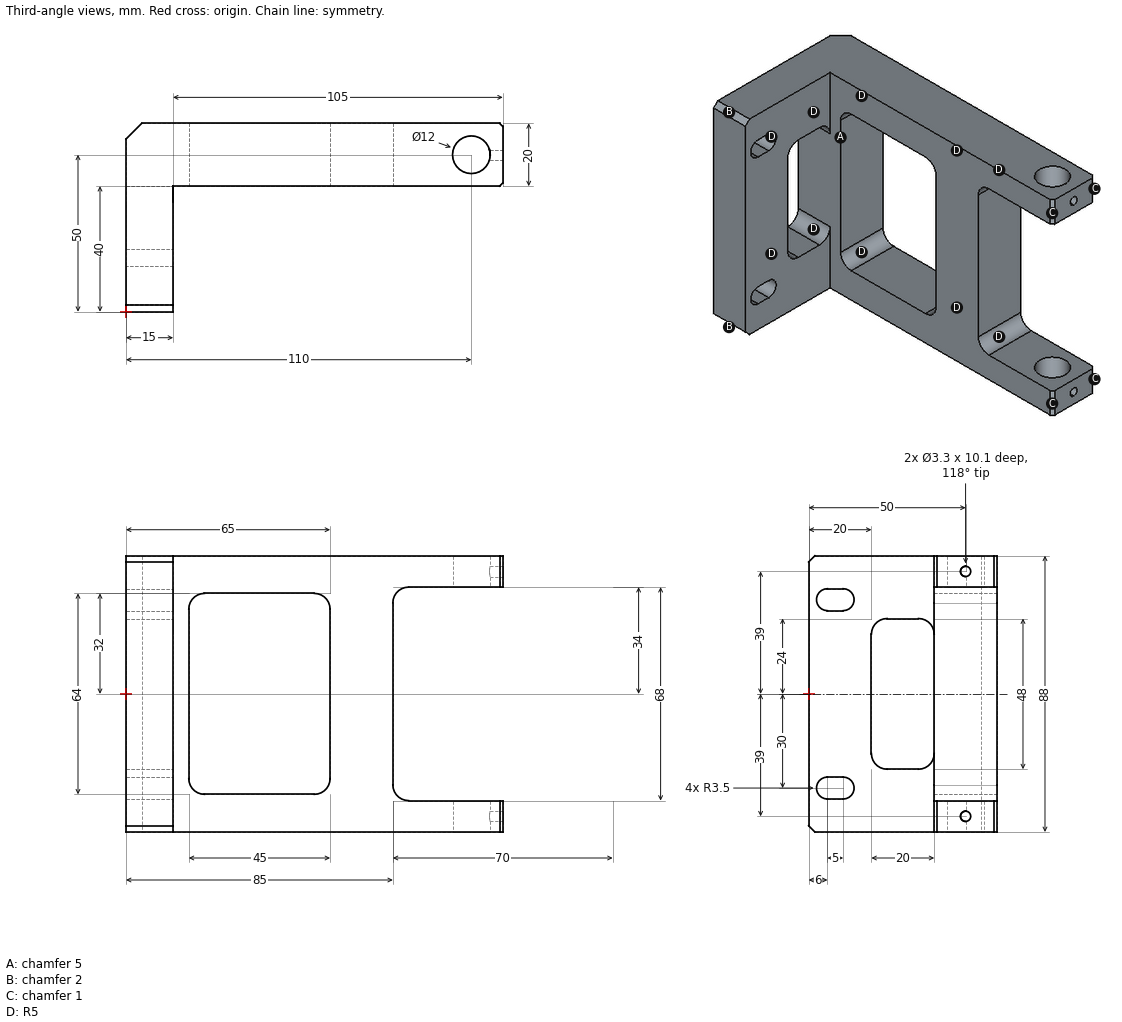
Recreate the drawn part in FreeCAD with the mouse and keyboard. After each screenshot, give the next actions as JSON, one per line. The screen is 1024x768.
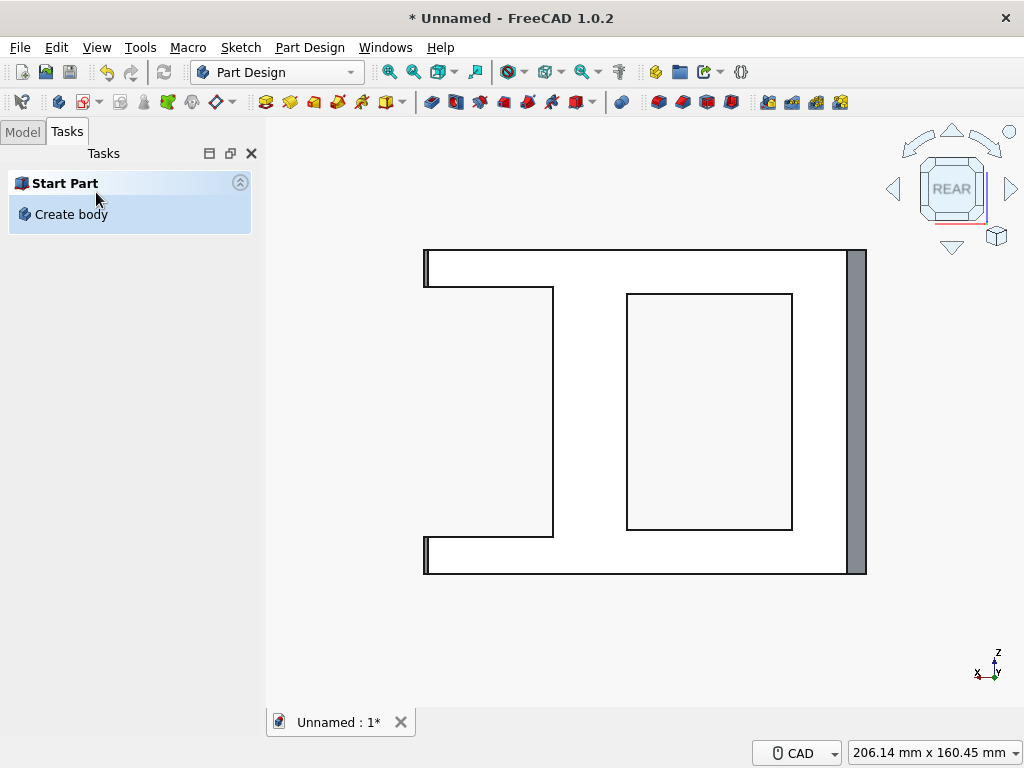
{"action": "key", "text": "6"}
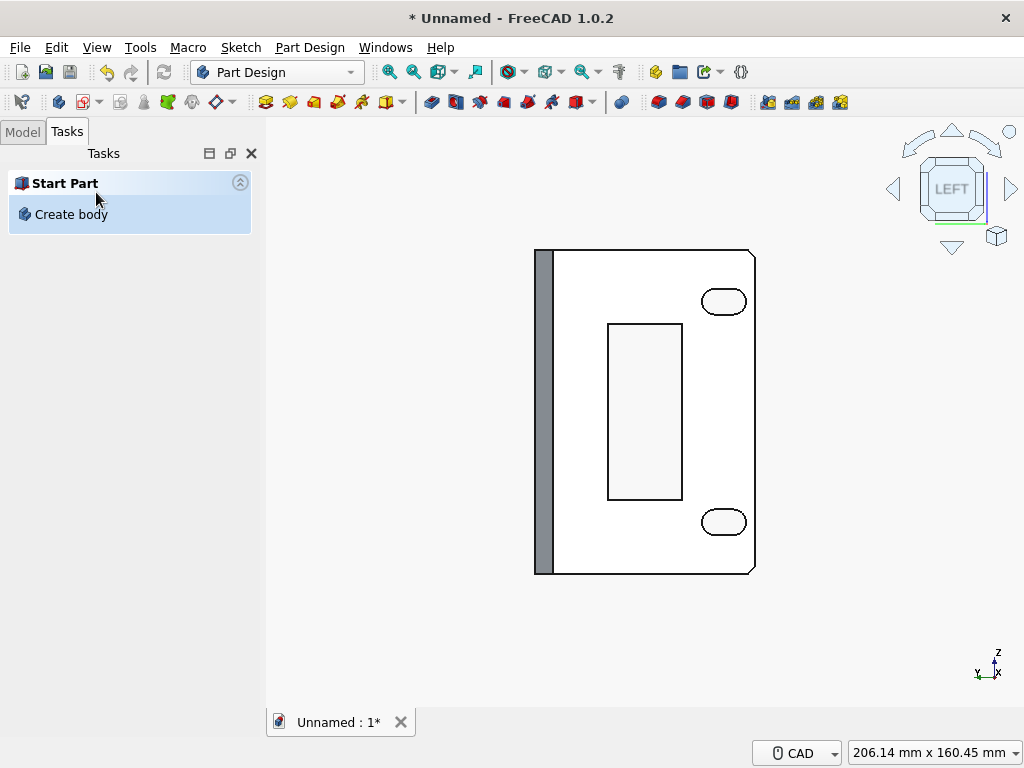
{"action": "key", "text": "v 3"}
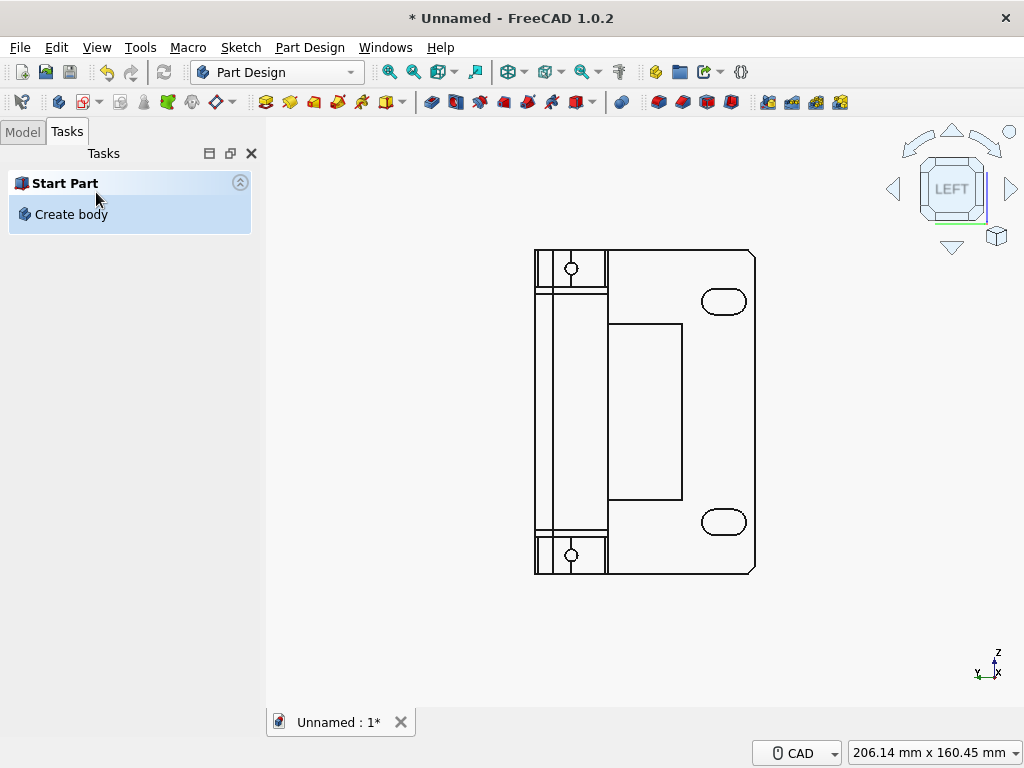
{"action": "key", "text": "0"}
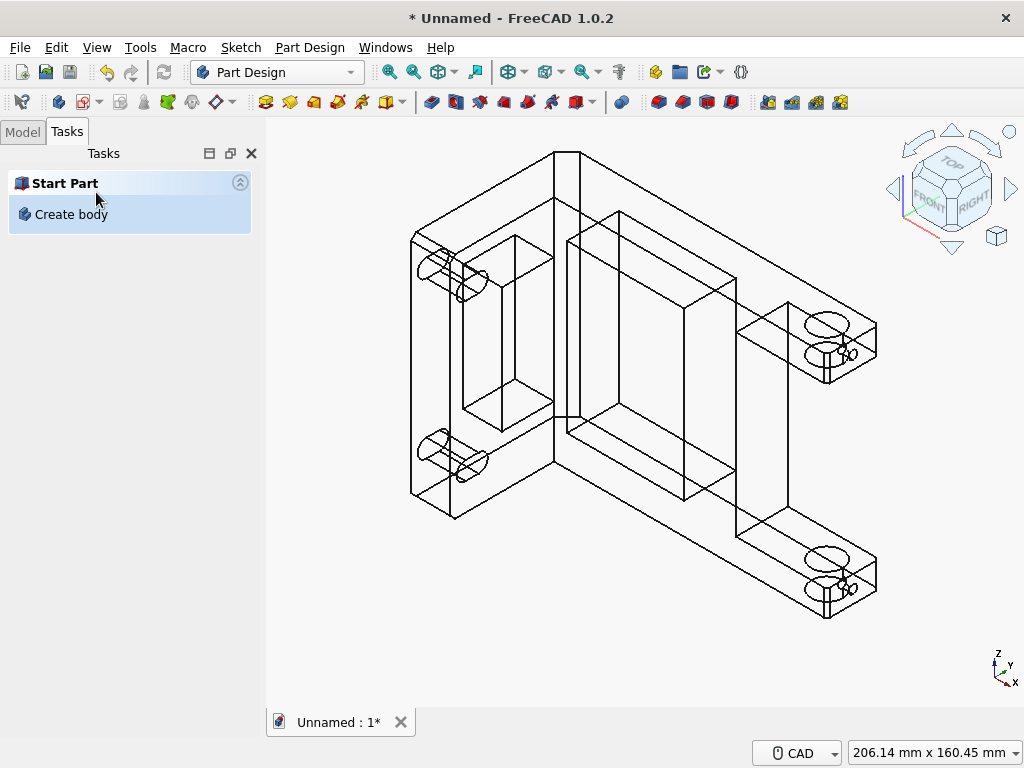
{"action": "left_click", "coordinate": [534, 245]}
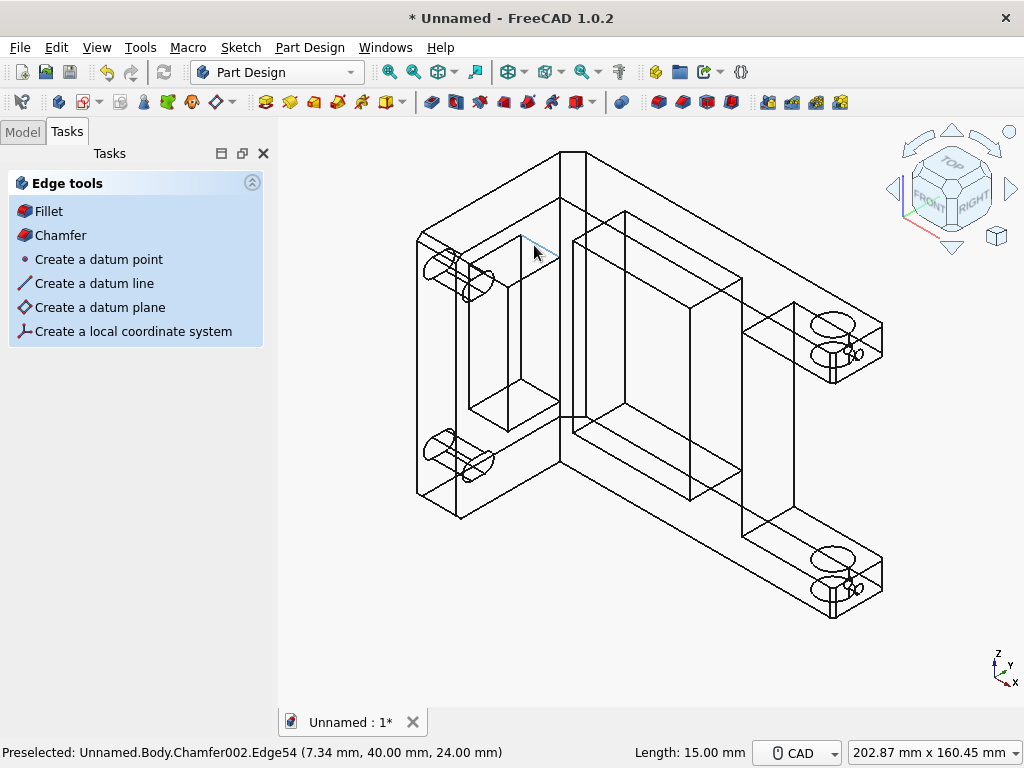
{"action": "left_click", "coordinate": [500, 282], "text": "ctrl"}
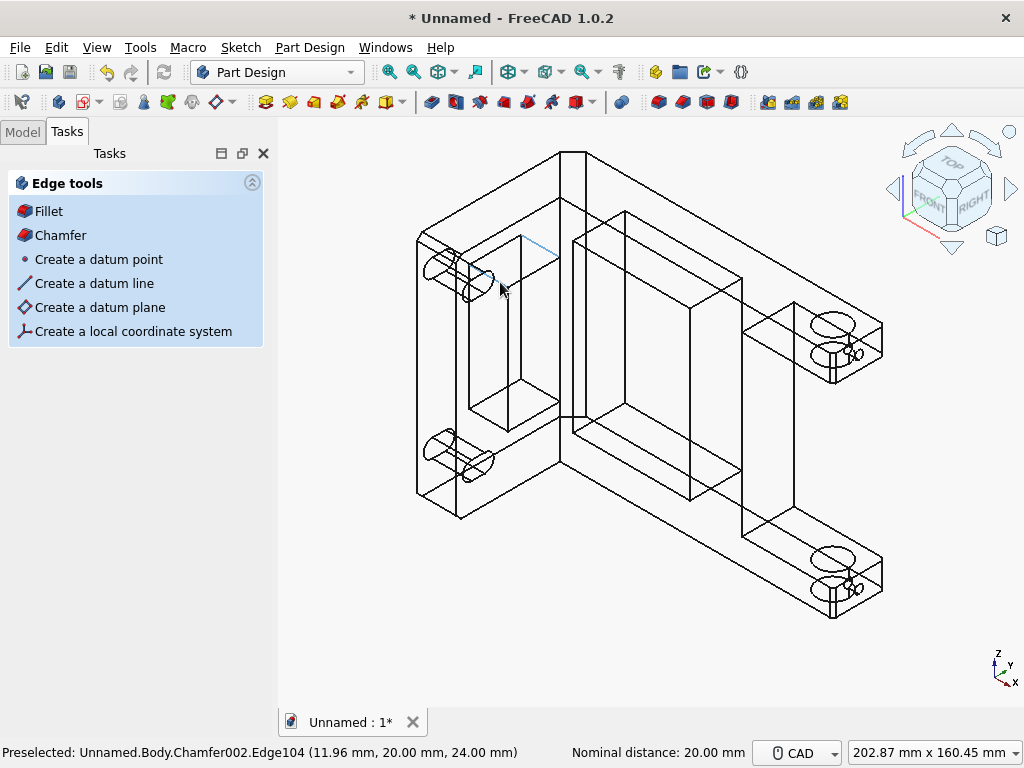
{"action": "left_click", "coordinate": [488, 419], "text": "ctrl"}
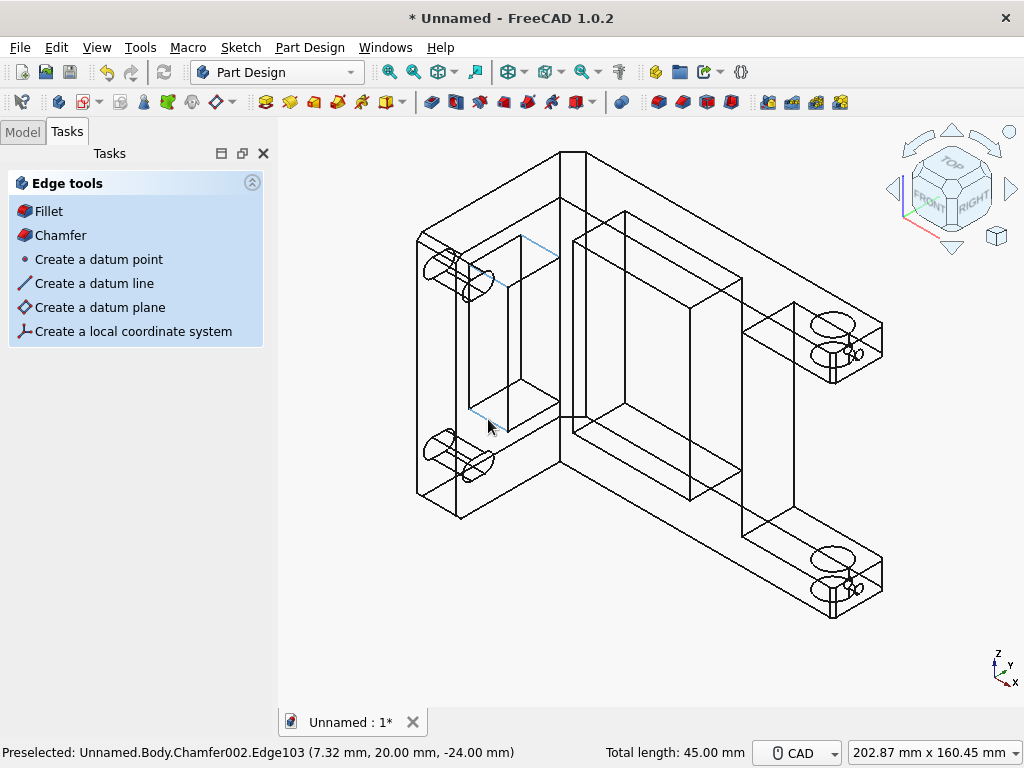
{"action": "left_click", "coordinate": [540, 389], "text": "ctrl"}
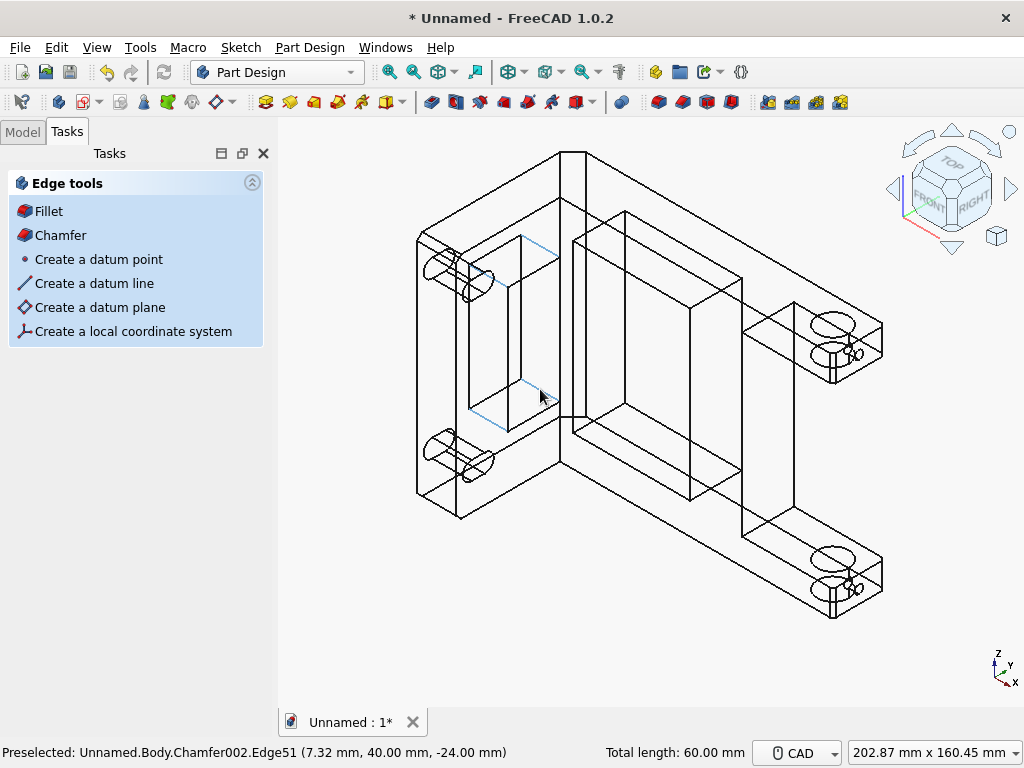
{"action": "left_click", "coordinate": [778, 310], "text": "ctrl"}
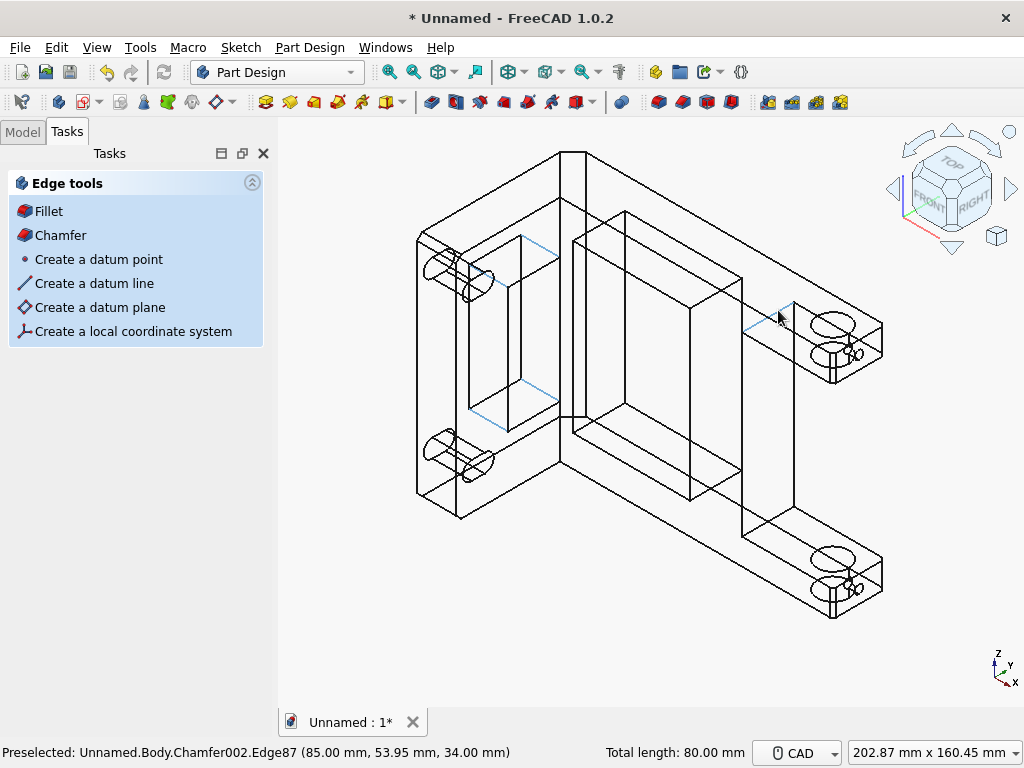
{"action": "left_click", "coordinate": [768, 521], "text": "ctrl"}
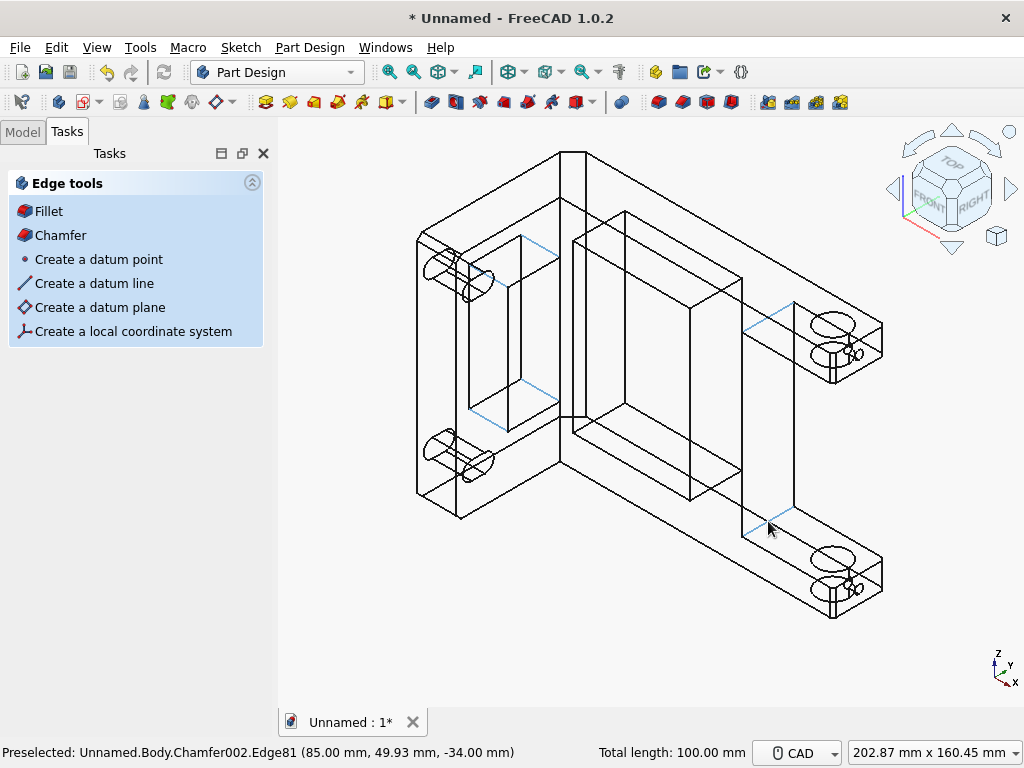
{"action": "left_click", "coordinate": [716, 485], "text": "ctrl"}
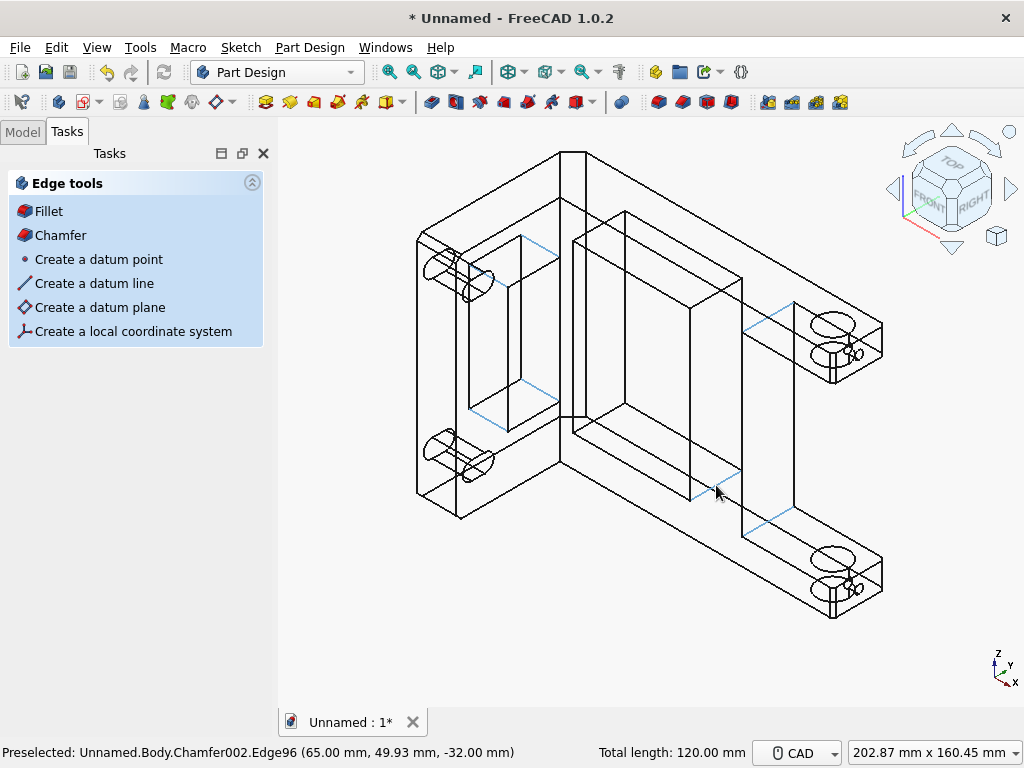
{"action": "left_click", "coordinate": [711, 295], "text": "ctrl"}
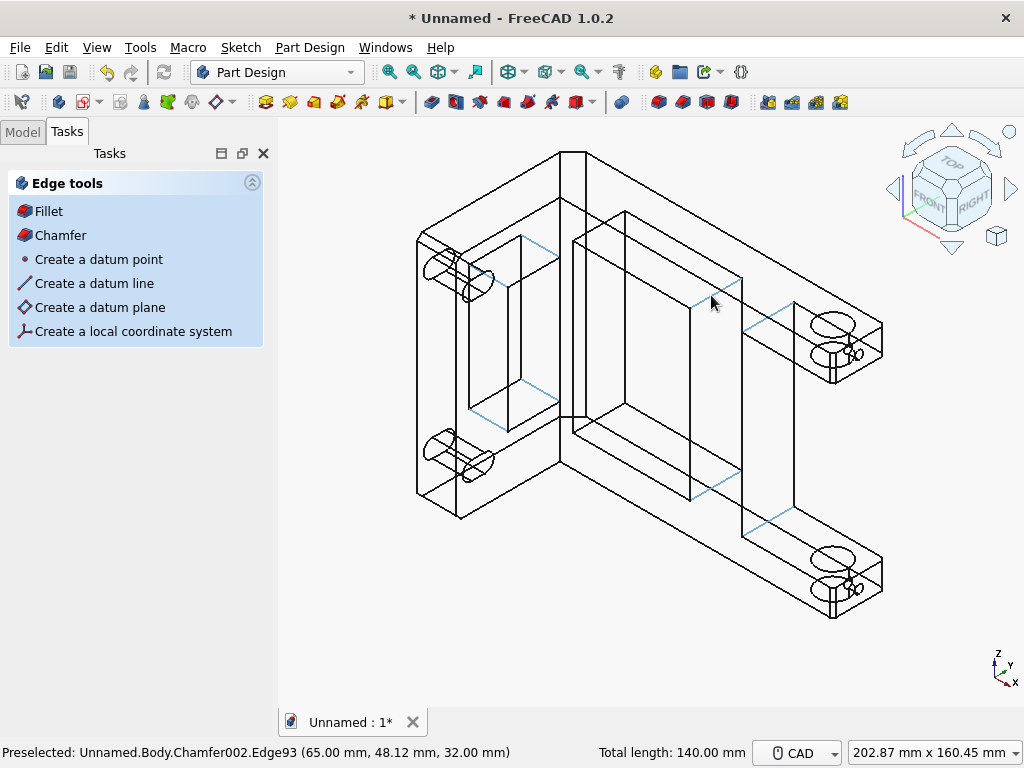
{"action": "left_click", "coordinate": [594, 228], "text": "ctrl"}